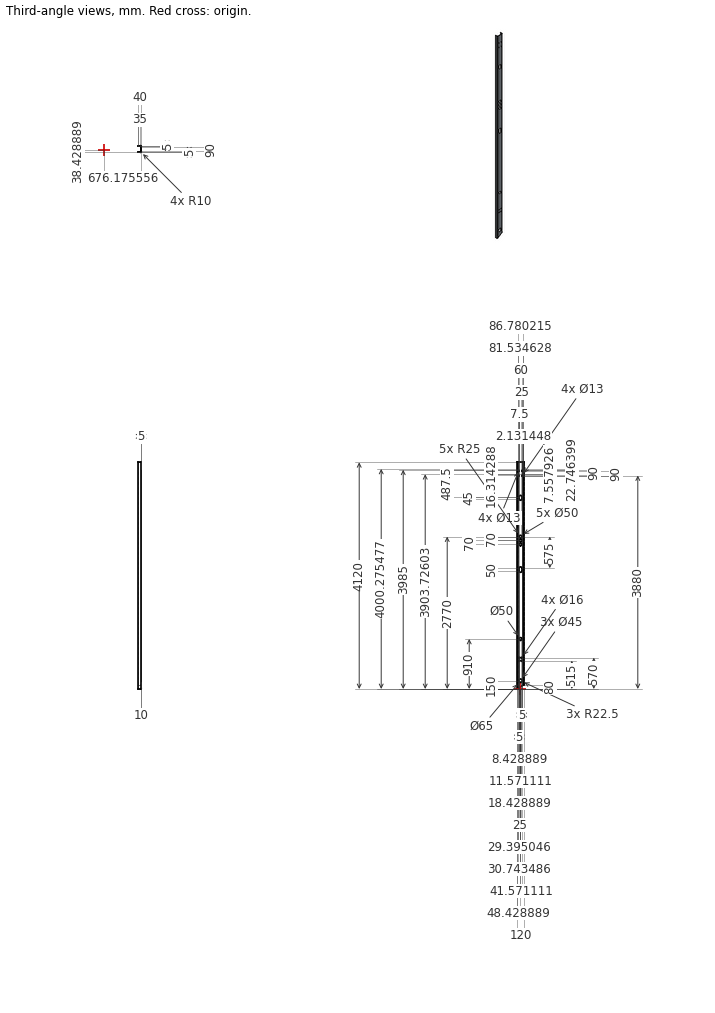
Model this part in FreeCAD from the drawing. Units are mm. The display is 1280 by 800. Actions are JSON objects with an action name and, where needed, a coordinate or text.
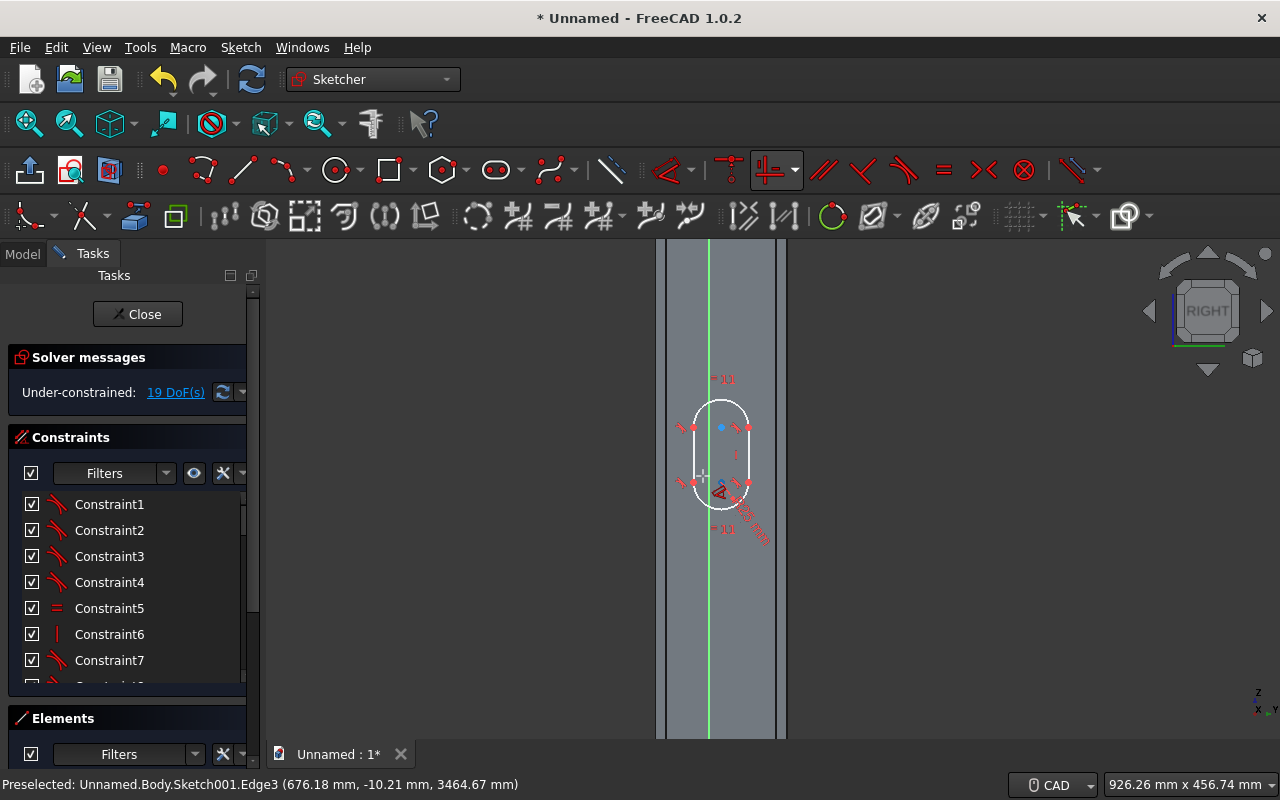
{"action": "left_click", "coordinate": [694, 466]}
{"action": "left_click", "coordinate": [660, 455]}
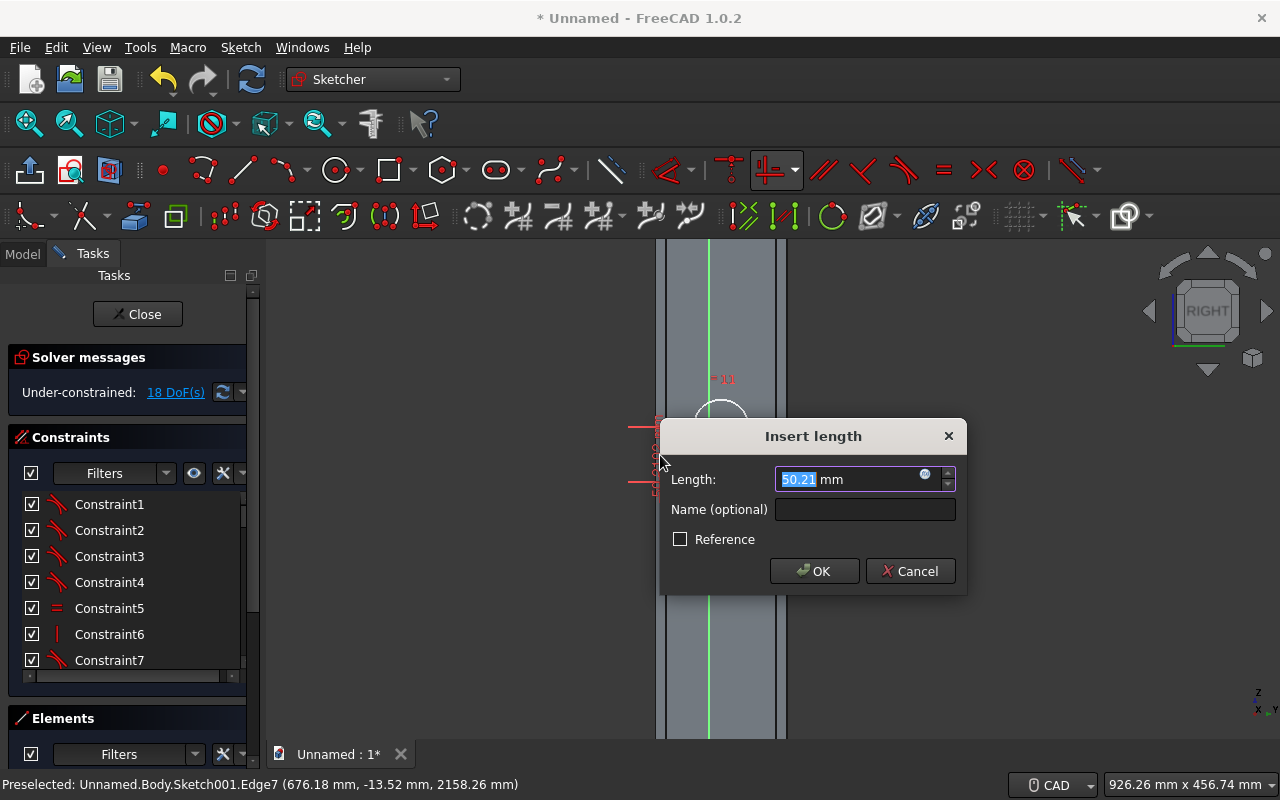
{"action": "type", "text": "50"}
{"action": "key", "text": "Return"}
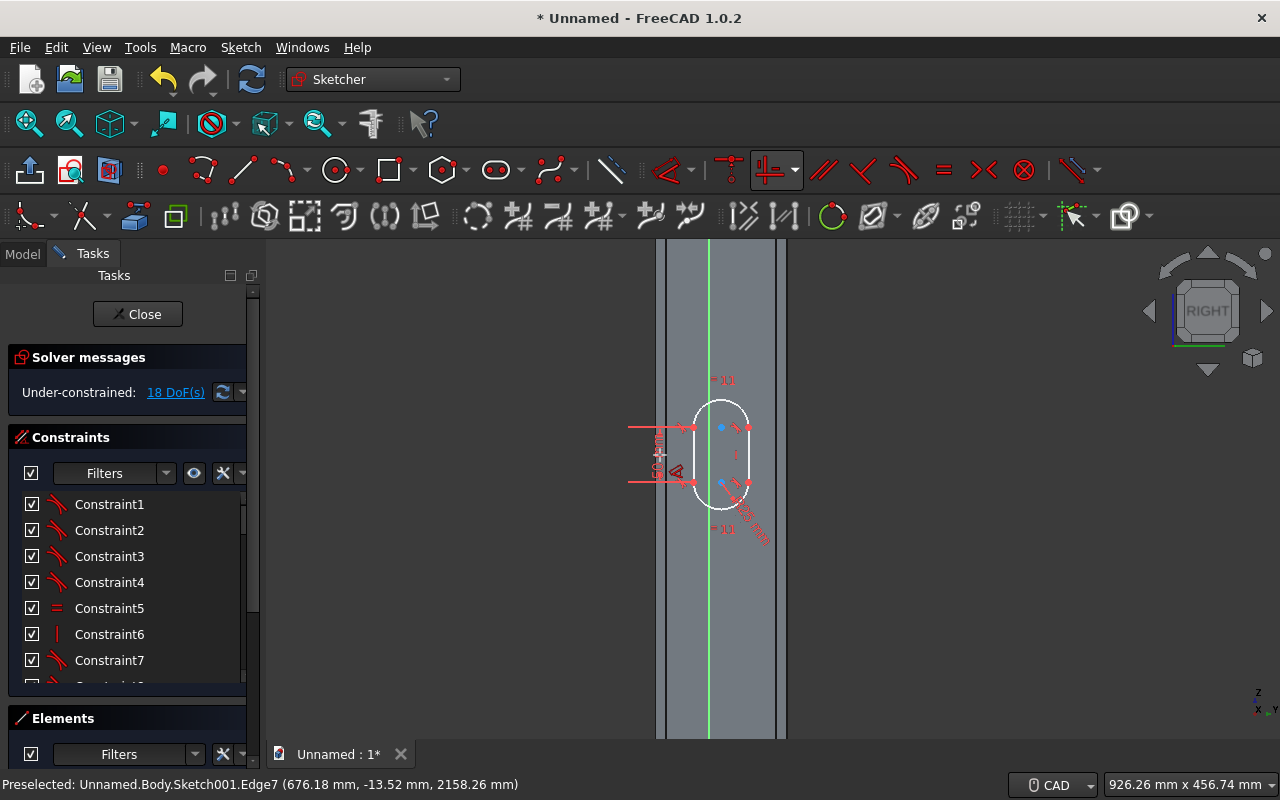
{"action": "scroll", "coordinate": [749, 482], "scroll_direction": "up", "scroll_amount": 10}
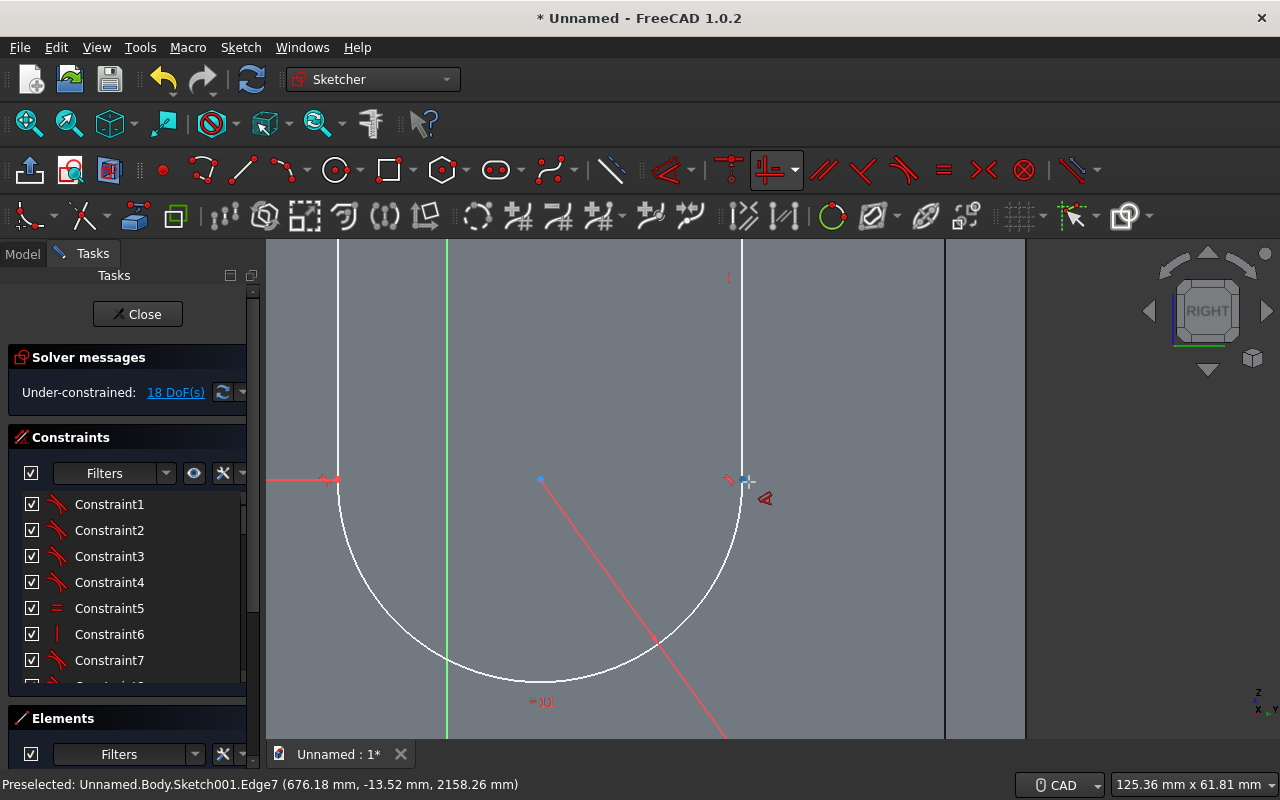
{"action": "left_click", "coordinate": [742, 480]}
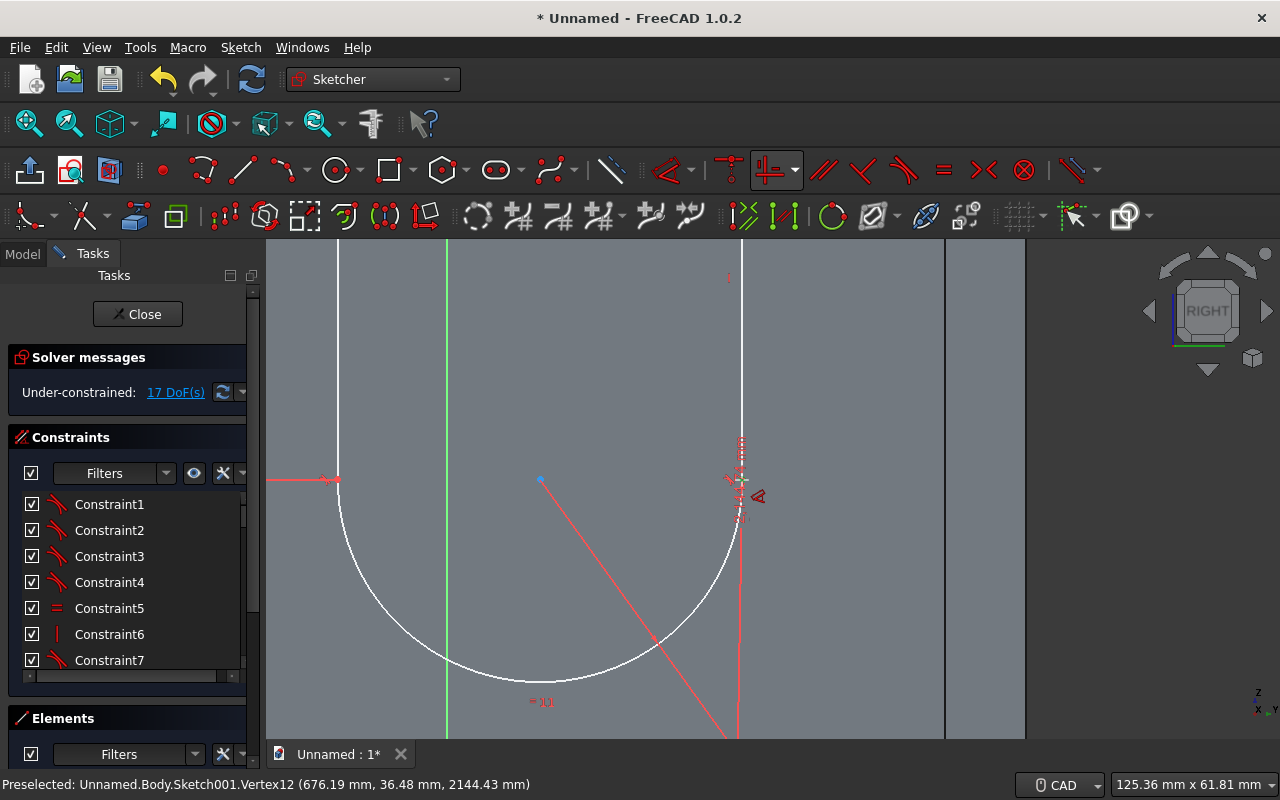
{"action": "scroll", "coordinate": [704, 489], "scroll_direction": "down", "scroll_amount": 15}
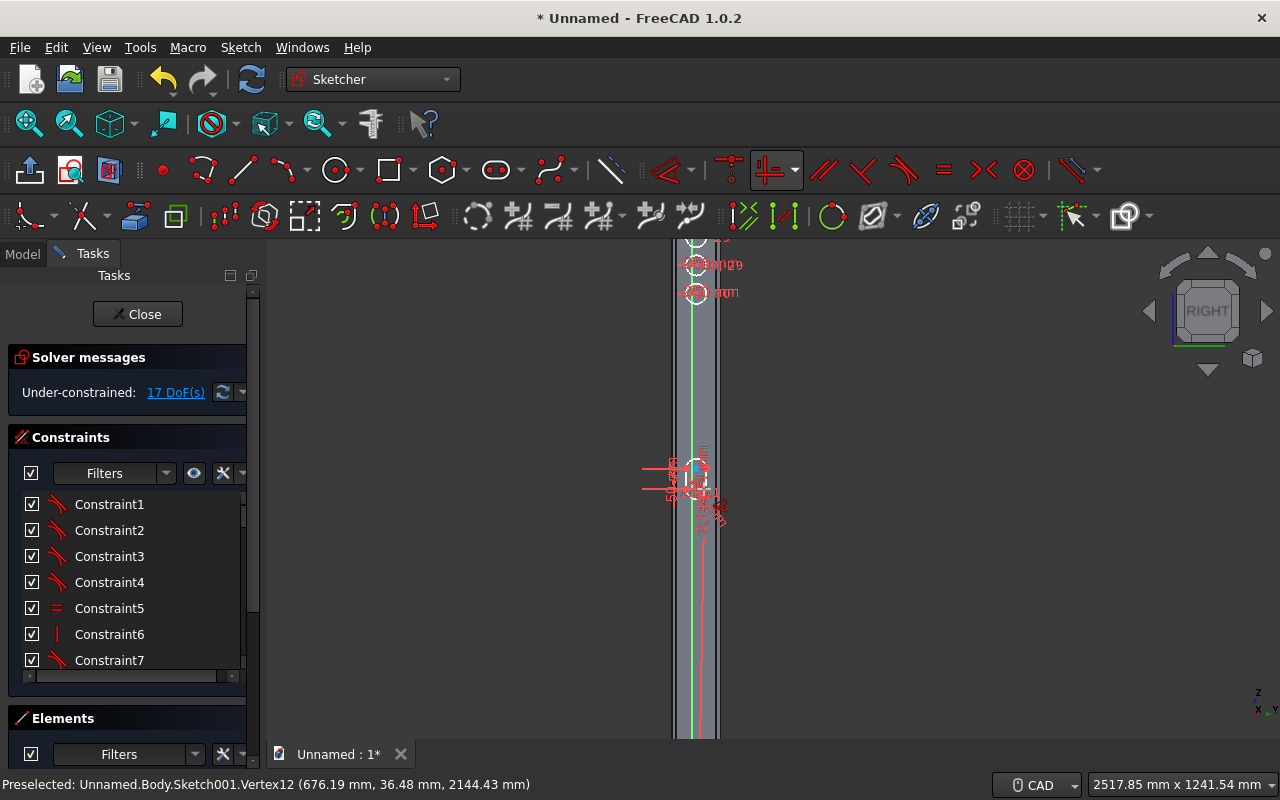
{"action": "scroll", "coordinate": [707, 474], "scroll_direction": "down", "scroll_amount": 8}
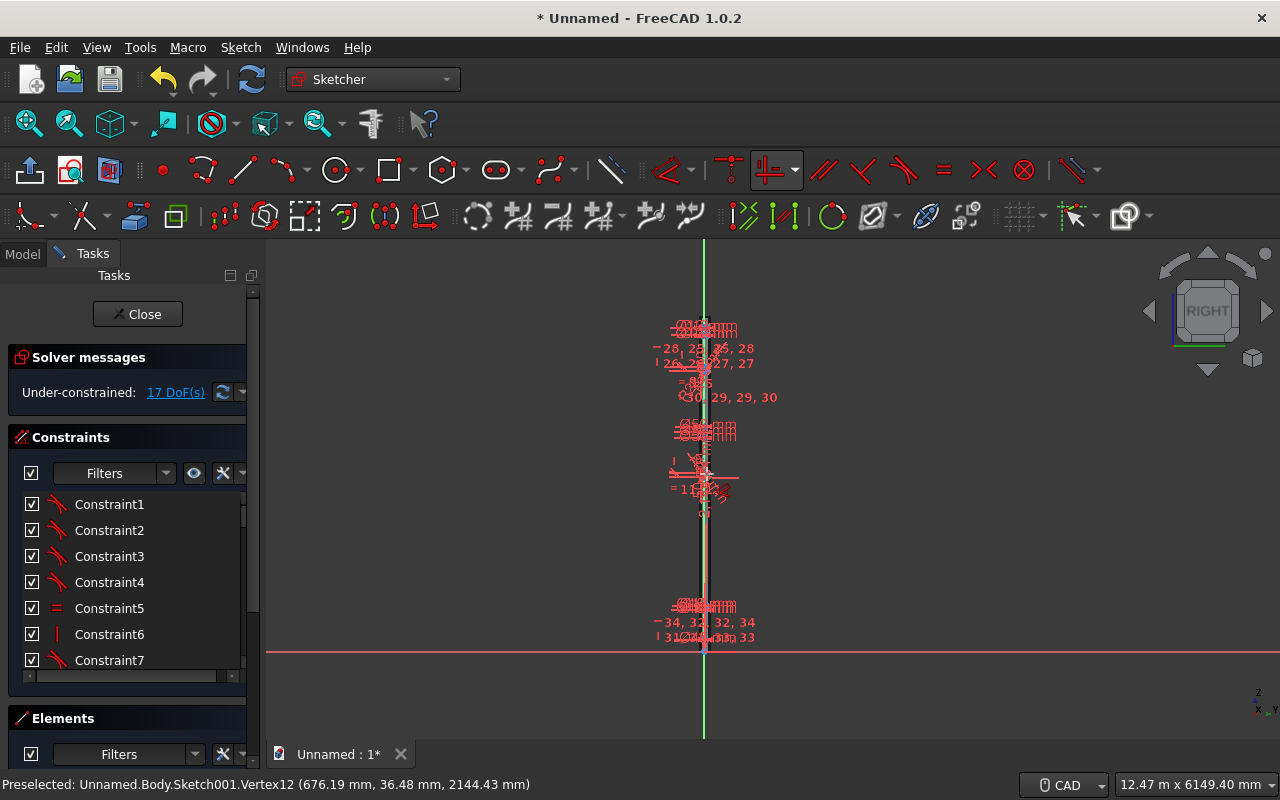
{"action": "scroll", "coordinate": [707, 606], "scroll_direction": "up", "scroll_amount": 23}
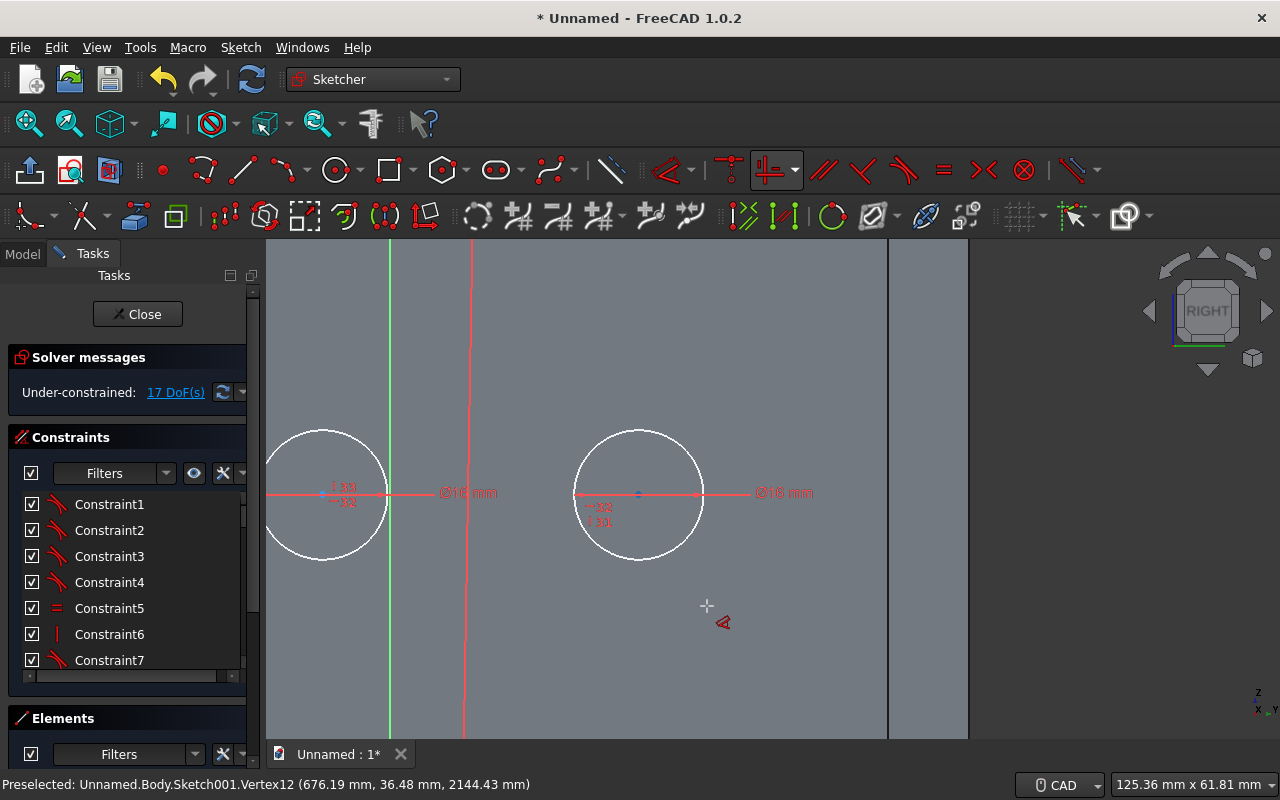
{"action": "left_click", "coordinate": [639, 495]}
{"action": "left_click", "coordinate": [662, 529]}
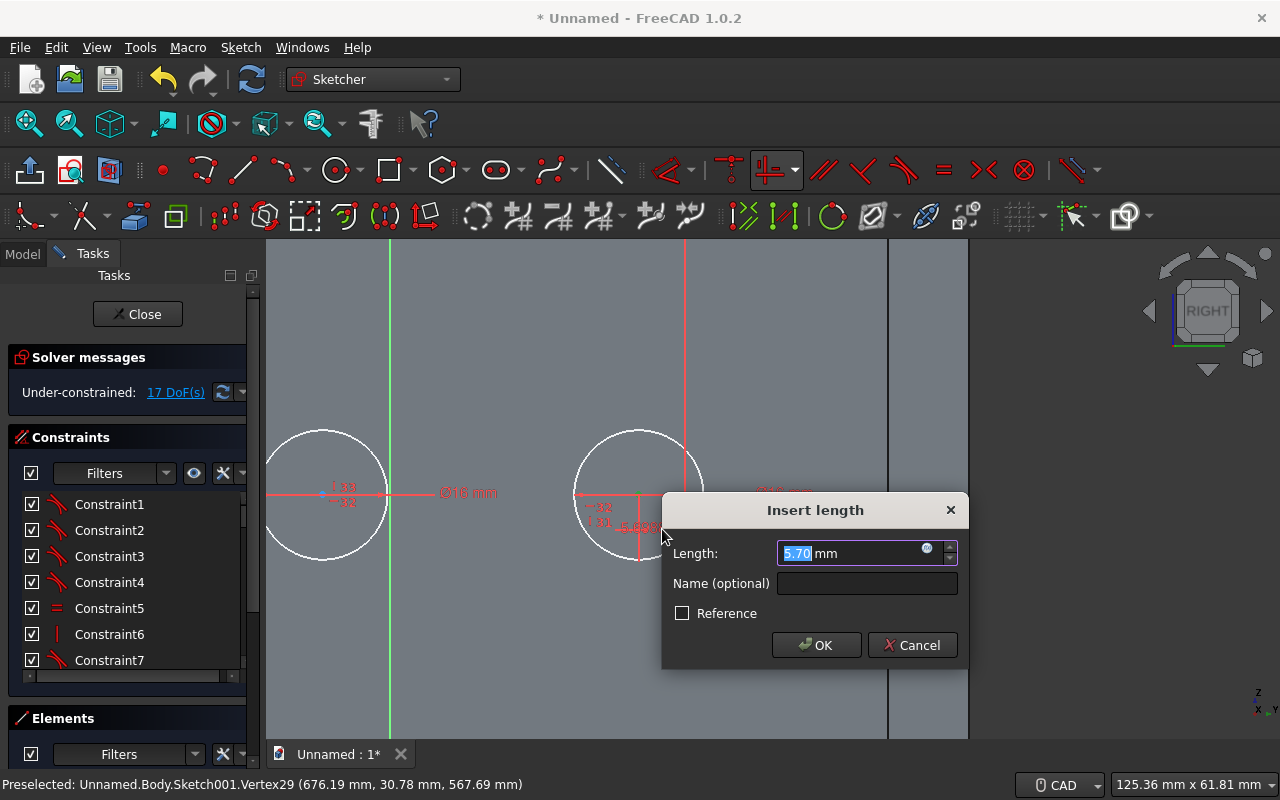
{"action": "type", "text": "5"}
{"action": "key", "text": "Return"}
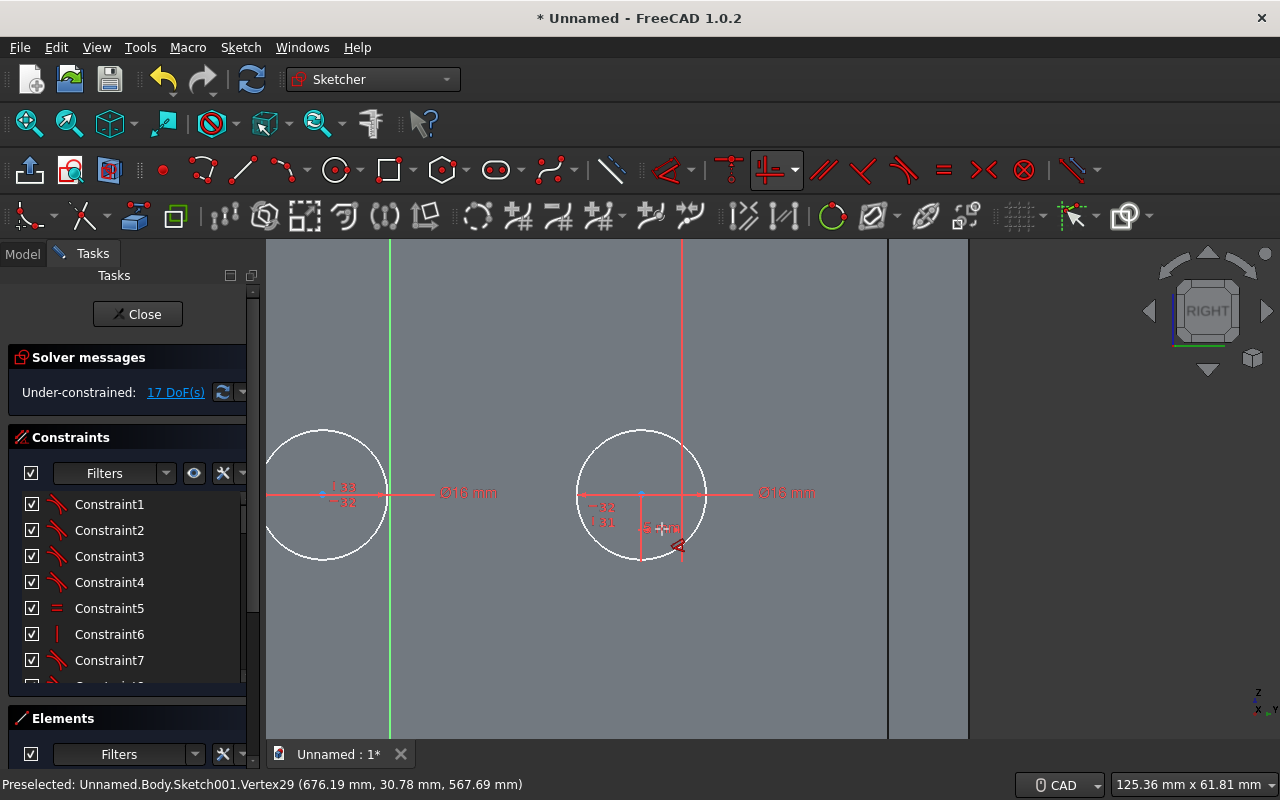
{"action": "scroll", "coordinate": [704, 489], "scroll_direction": "down", "scroll_amount": 15}